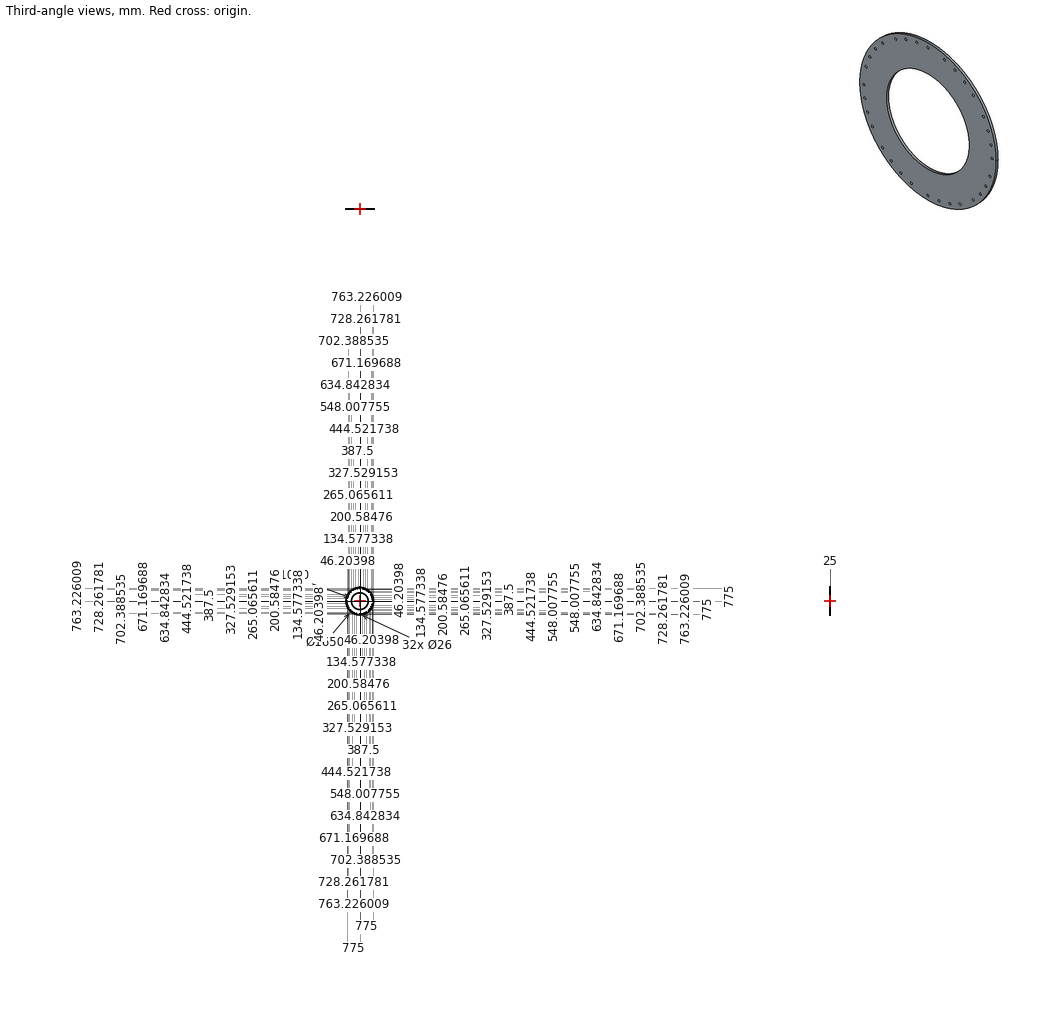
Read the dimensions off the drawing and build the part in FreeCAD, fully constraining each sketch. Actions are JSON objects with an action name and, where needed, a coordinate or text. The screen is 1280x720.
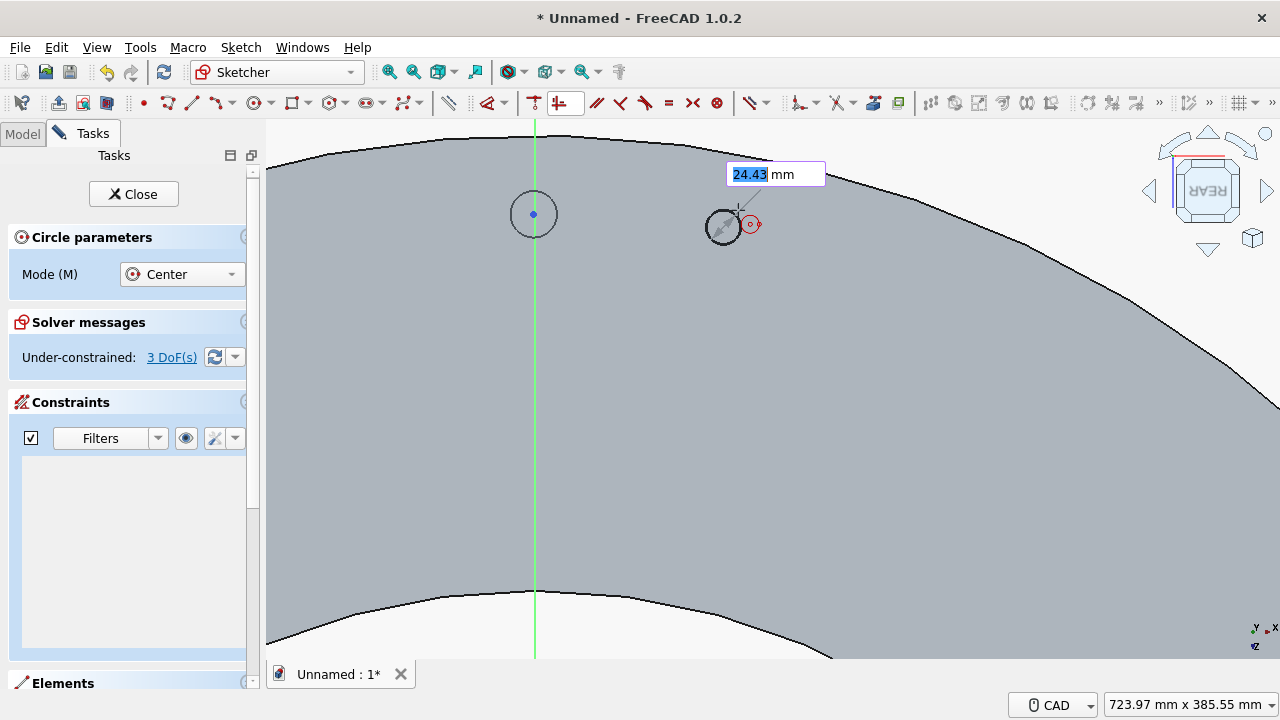
{"action": "left_click", "coordinate": [736, 209]}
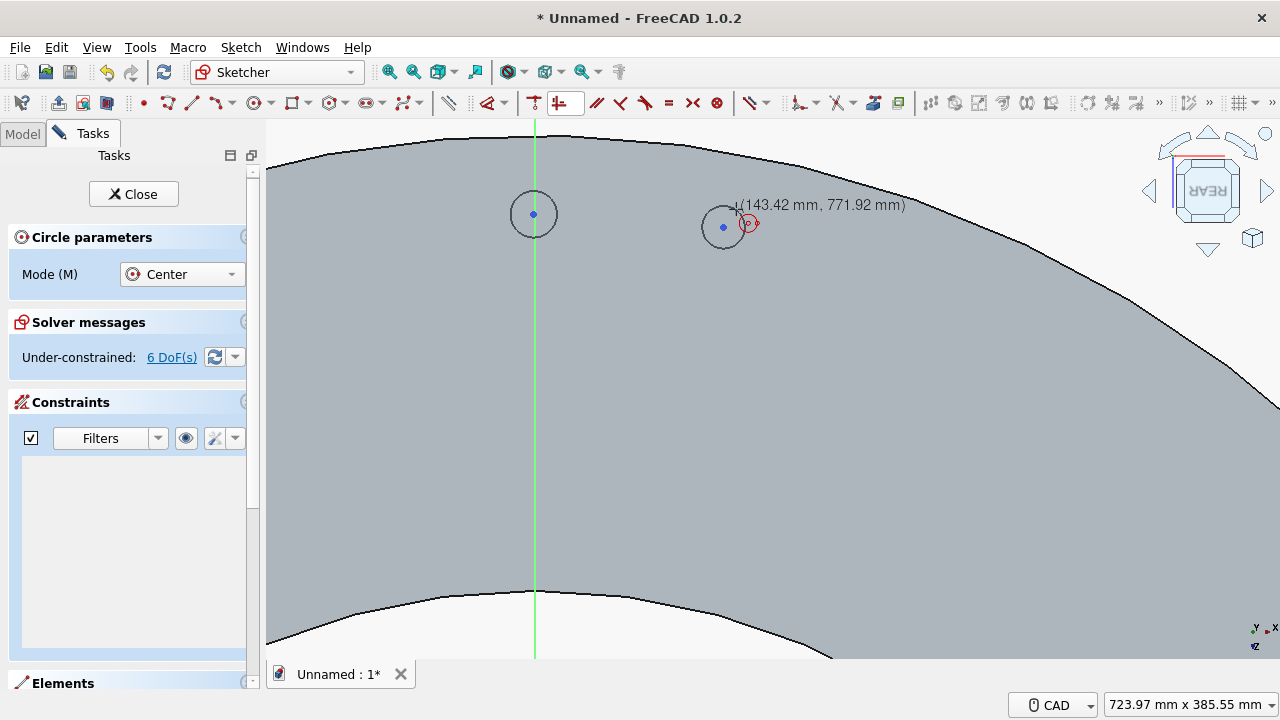
{"action": "scroll", "coordinate": [906, 271], "scroll_direction": "up", "scroll_amount": 2}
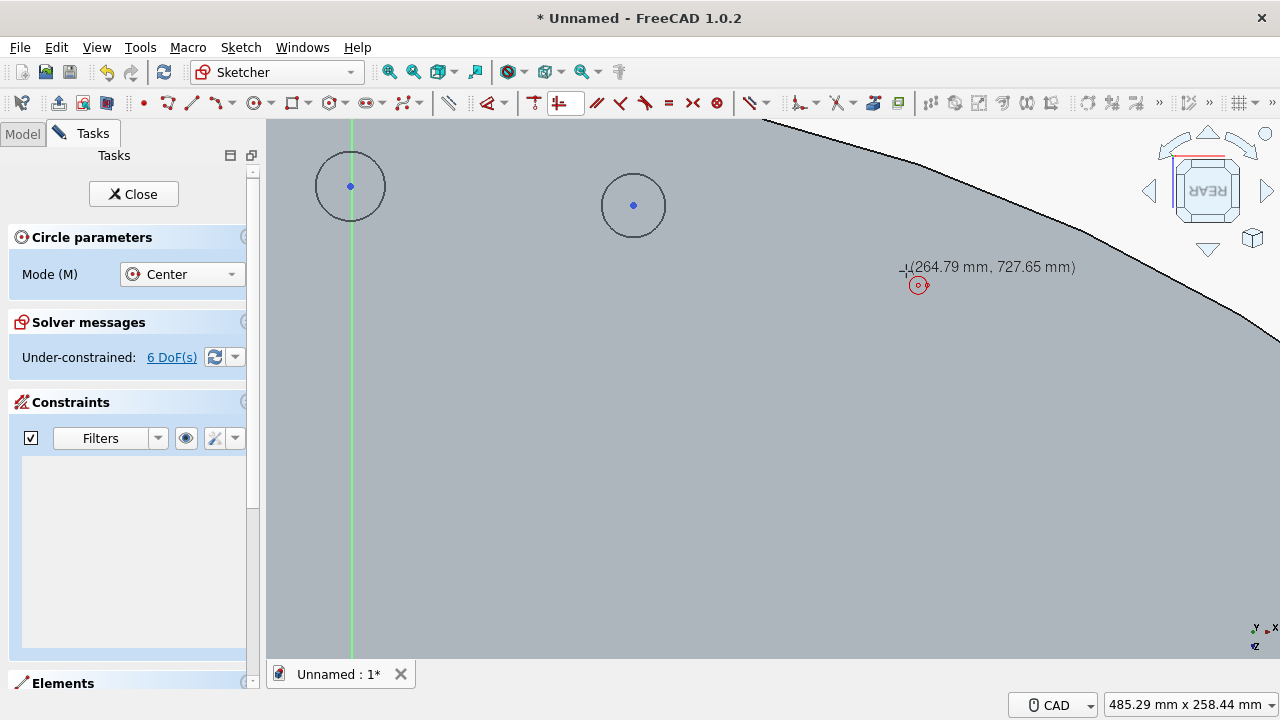
{"action": "scroll", "coordinate": [748, 214], "scroll_direction": "down", "scroll_amount": 11}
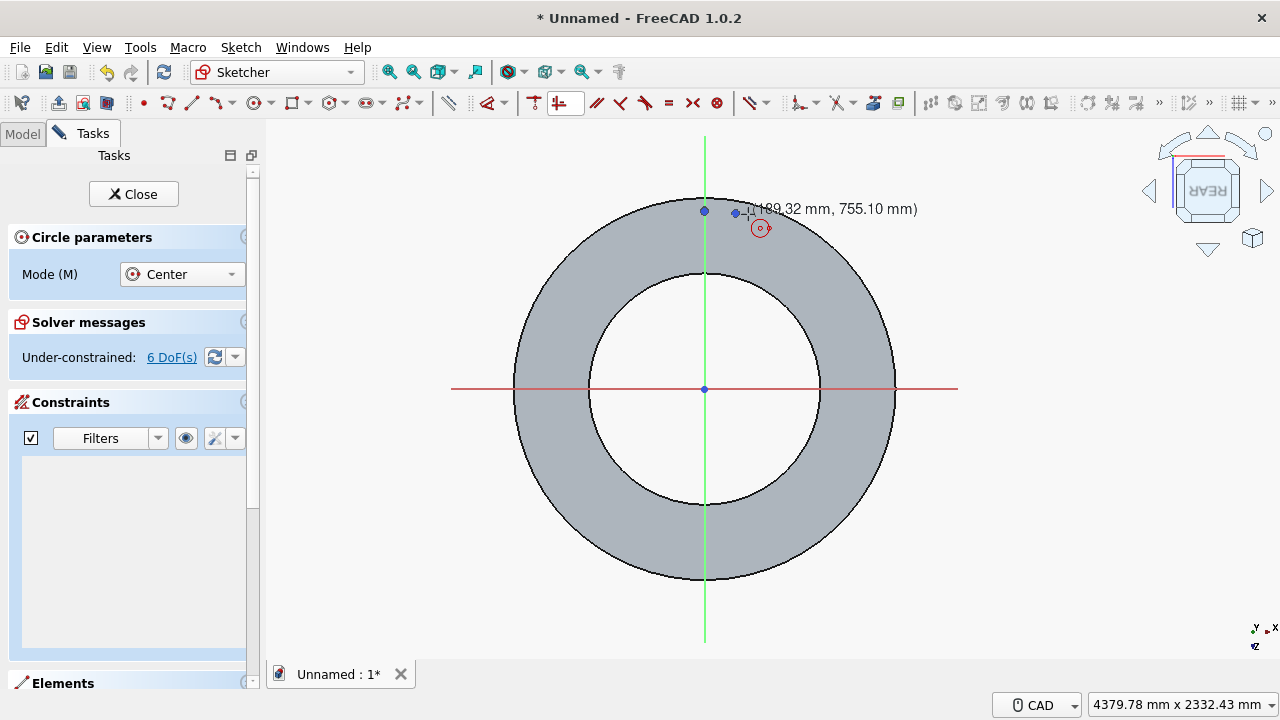
{"action": "left_click", "coordinate": [766, 220]}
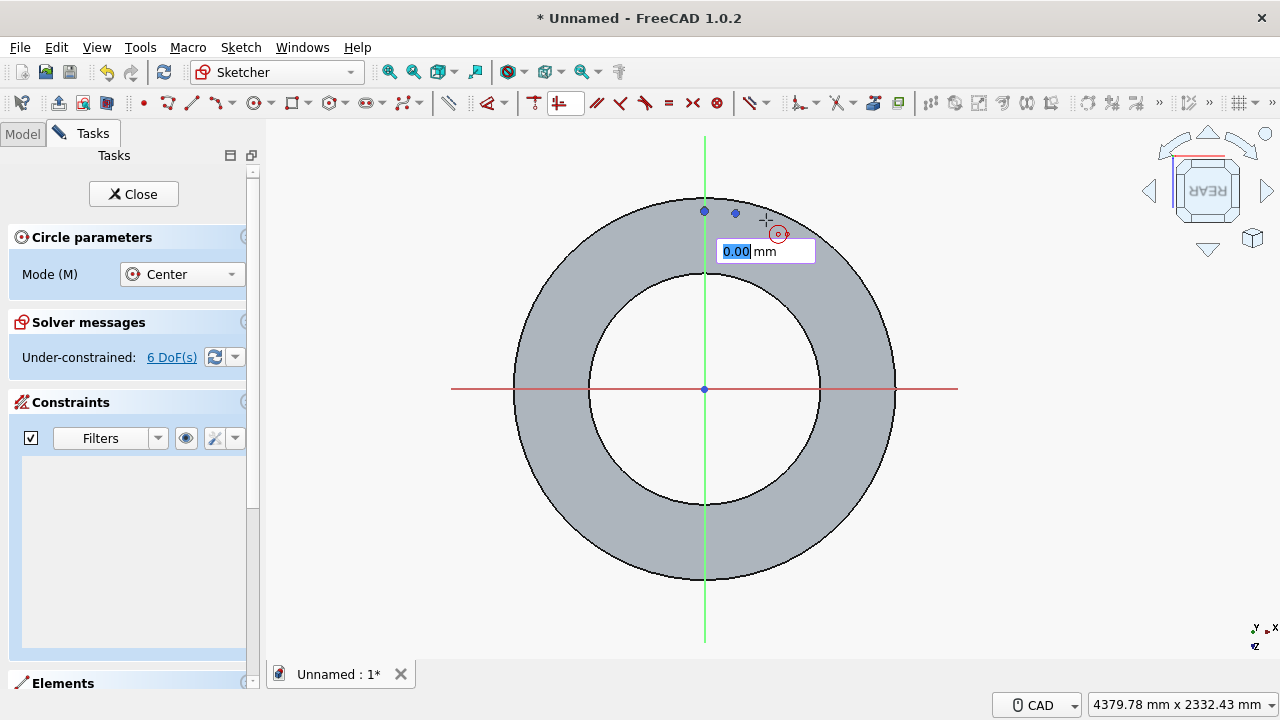
{"action": "scroll", "coordinate": [768, 218], "scroll_direction": "up", "scroll_amount": 9}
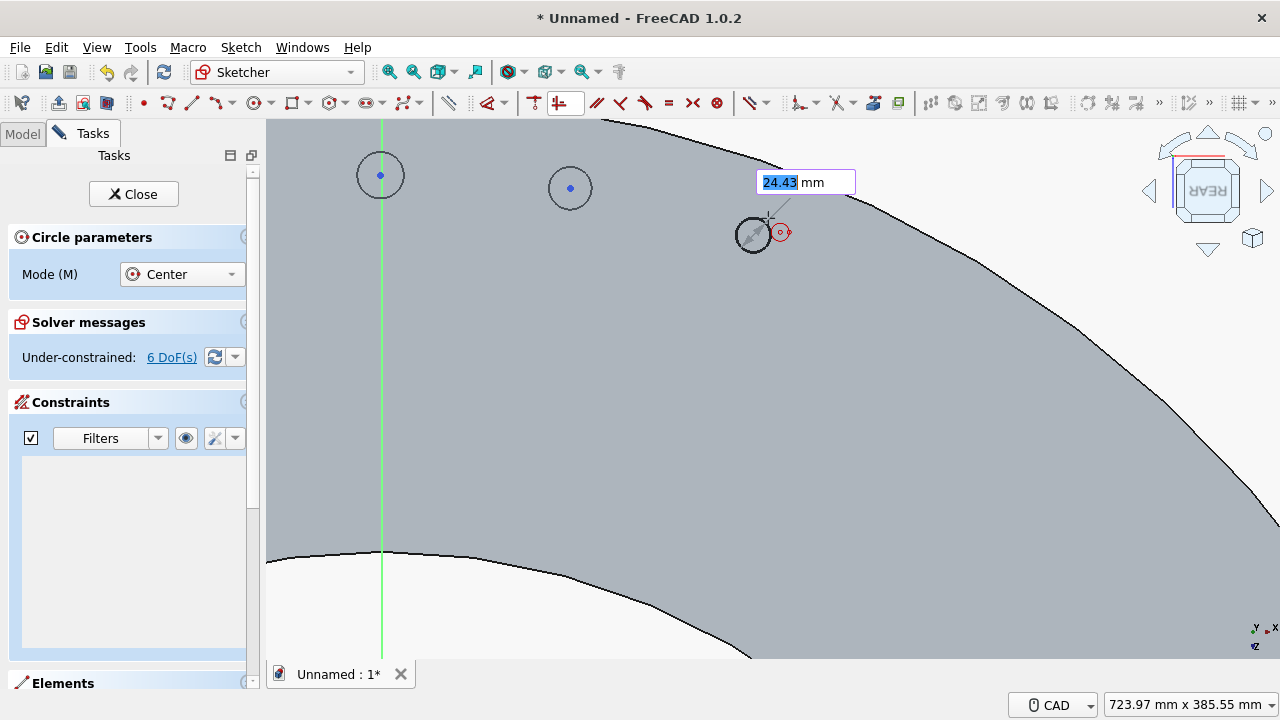
{"action": "left_click", "coordinate": [766, 219]}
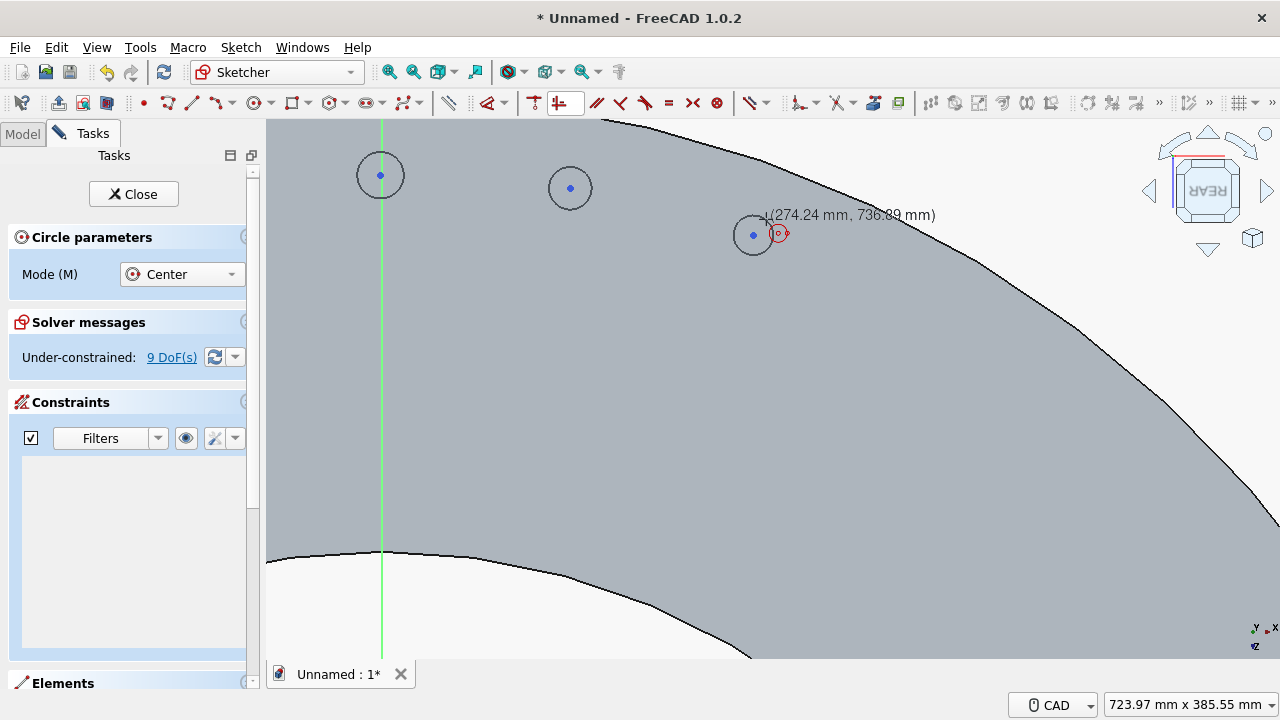
{"action": "scroll", "coordinate": [925, 312], "scroll_direction": "up", "scroll_amount": 2}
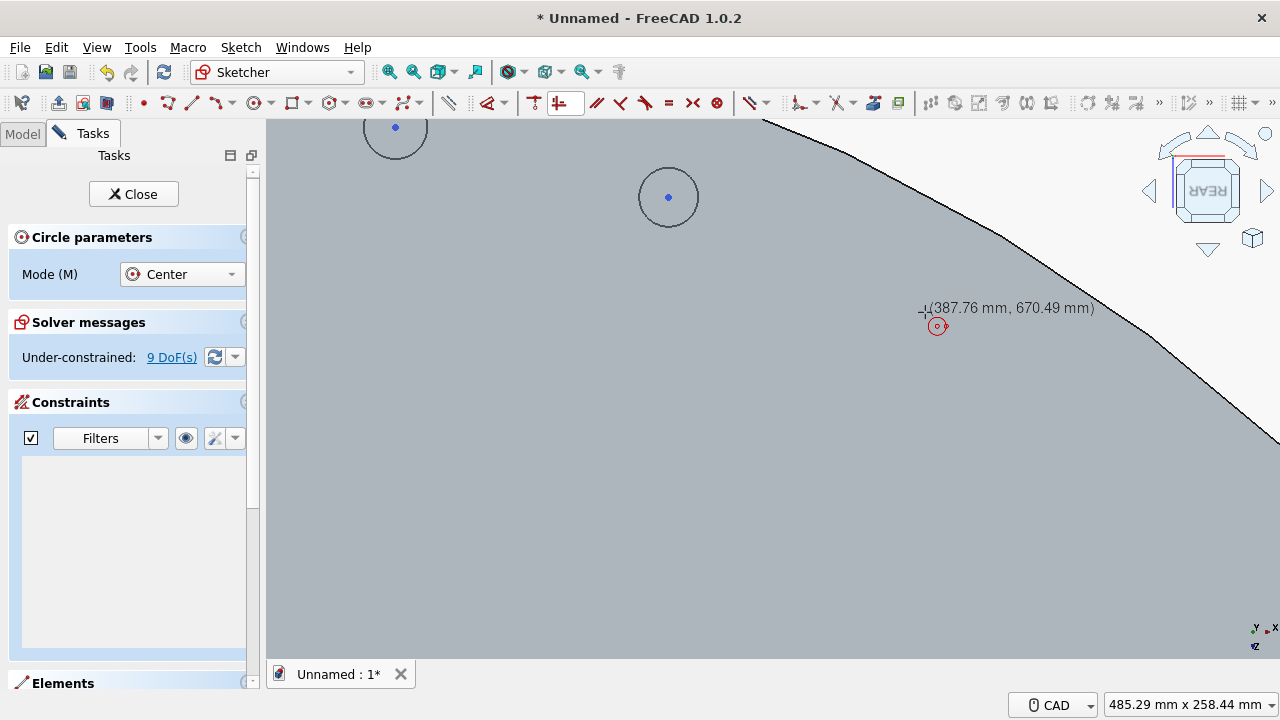
{"action": "scroll", "coordinate": [778, 224], "scroll_direction": "down", "scroll_amount": 11}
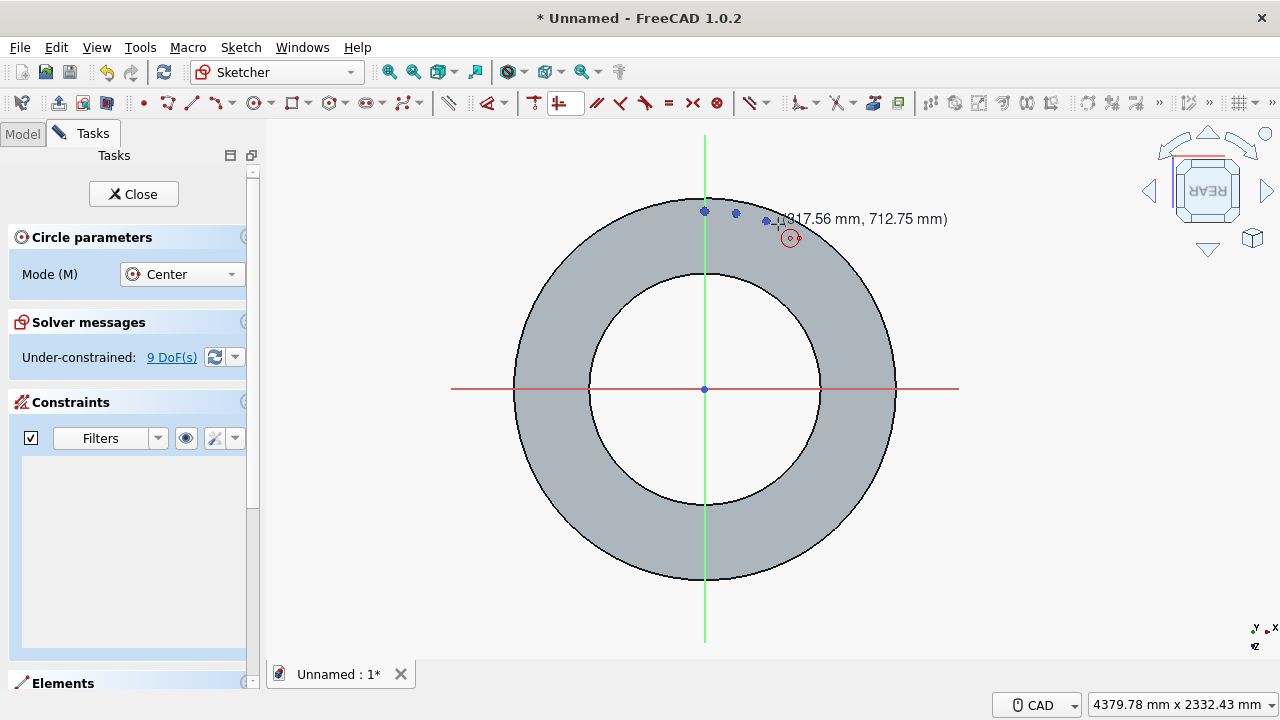
{"action": "left_click", "coordinate": [795, 234]}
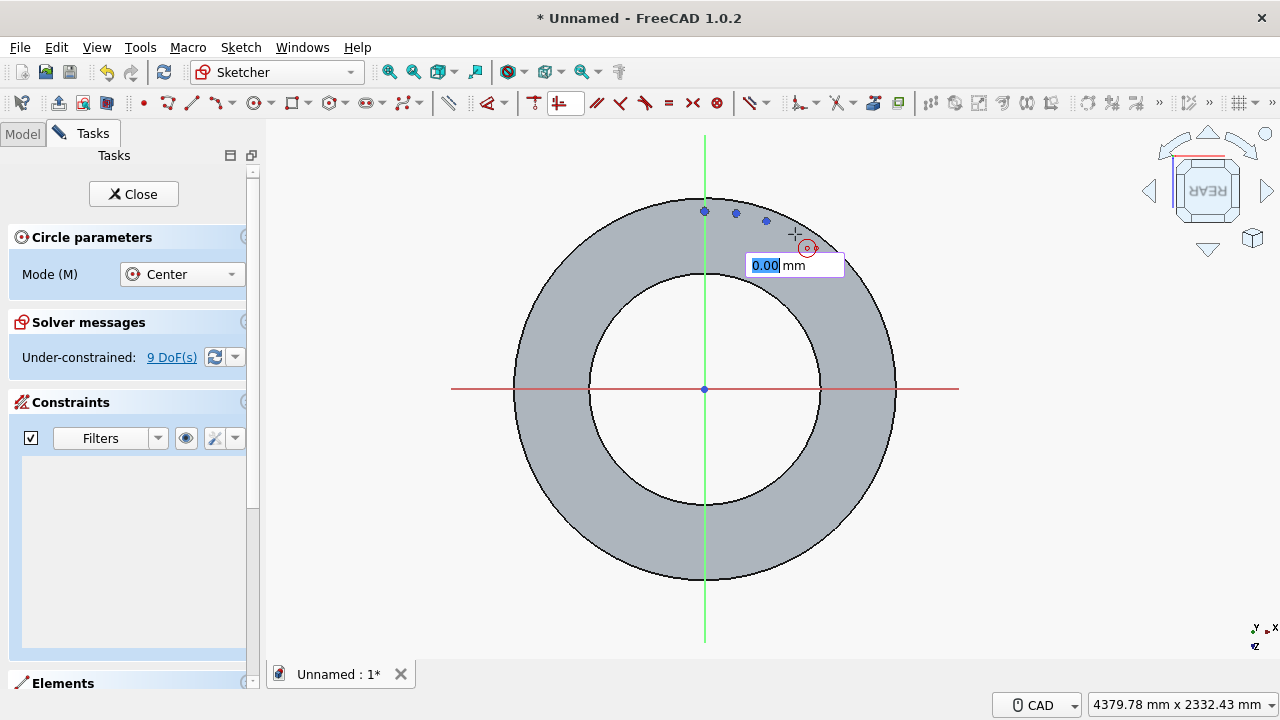
{"action": "scroll", "coordinate": [797, 232], "scroll_direction": "up", "scroll_amount": 9}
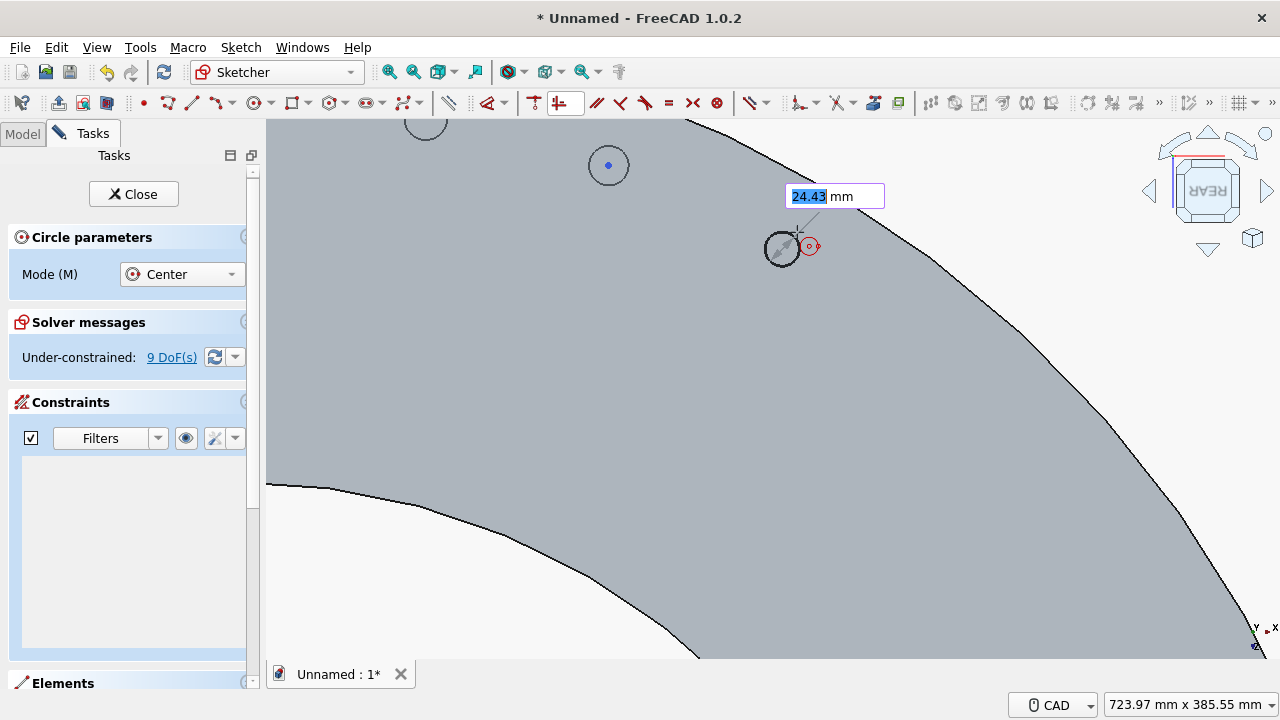
{"action": "left_click", "coordinate": [793, 230]}